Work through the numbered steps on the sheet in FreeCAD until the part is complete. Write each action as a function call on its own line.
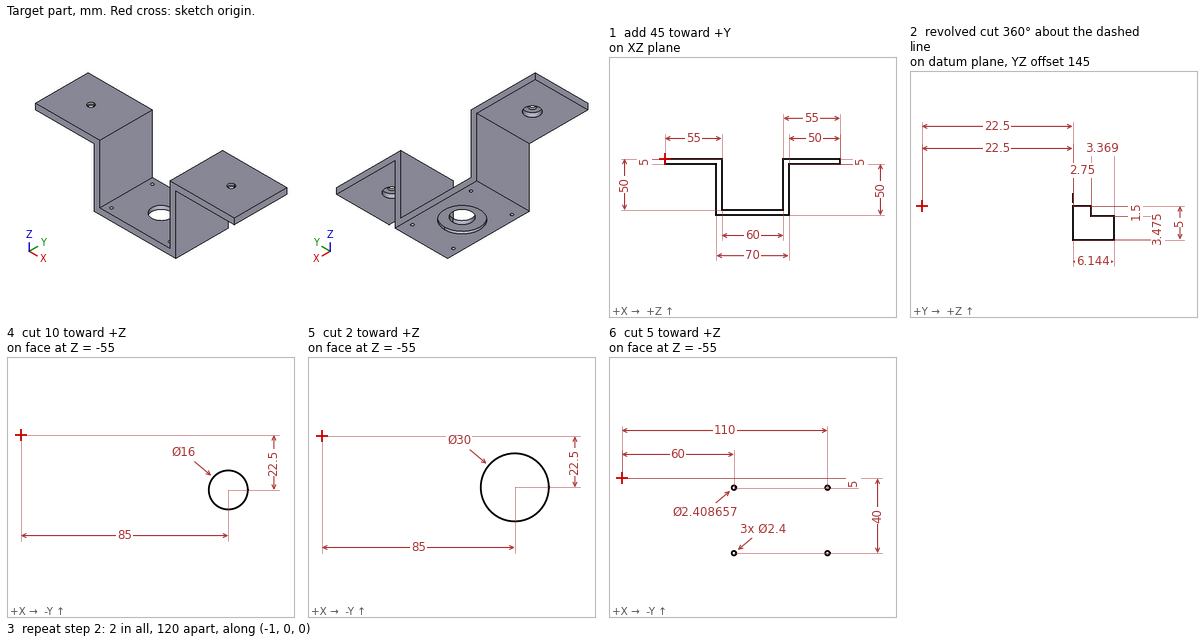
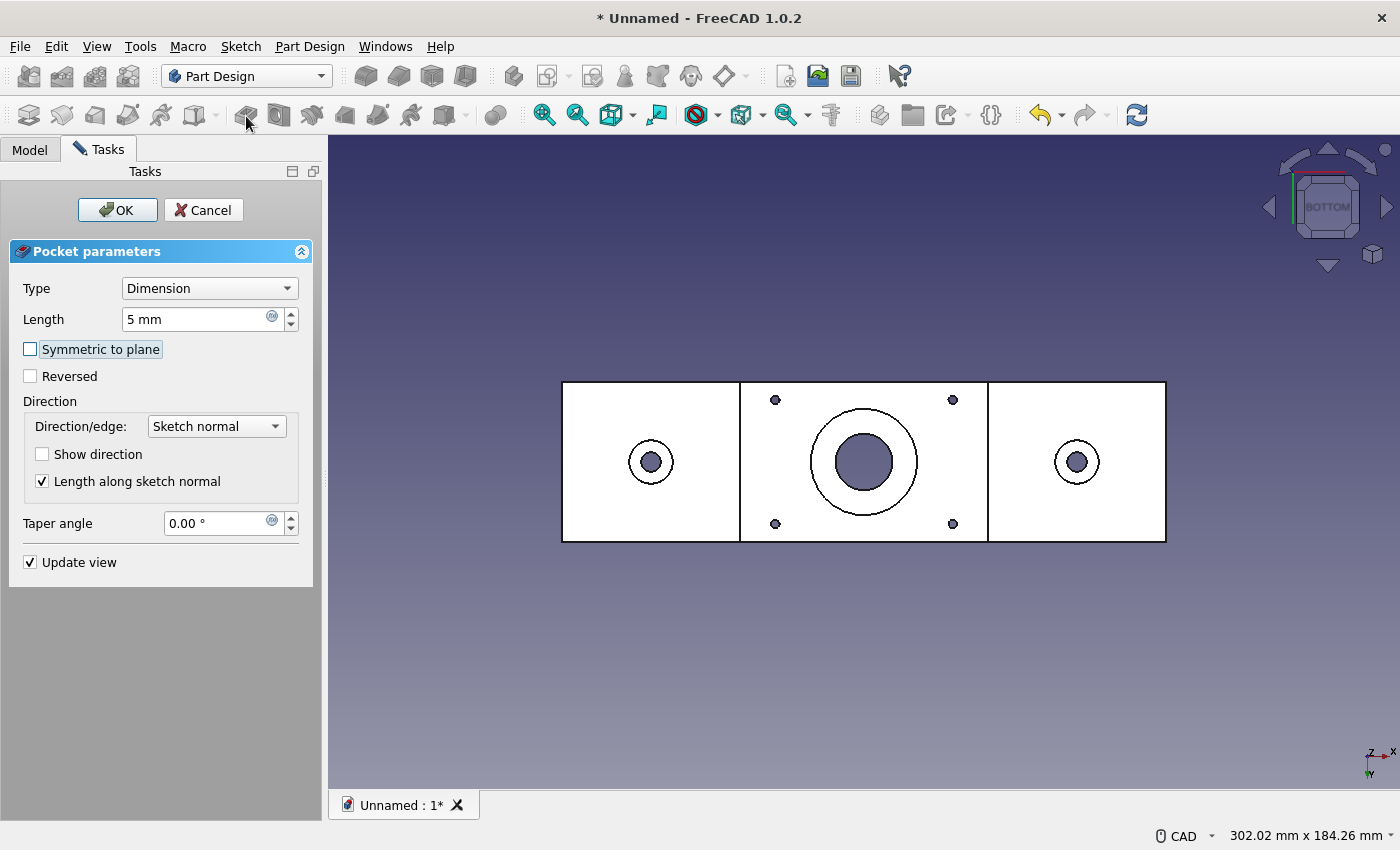
click(118, 210)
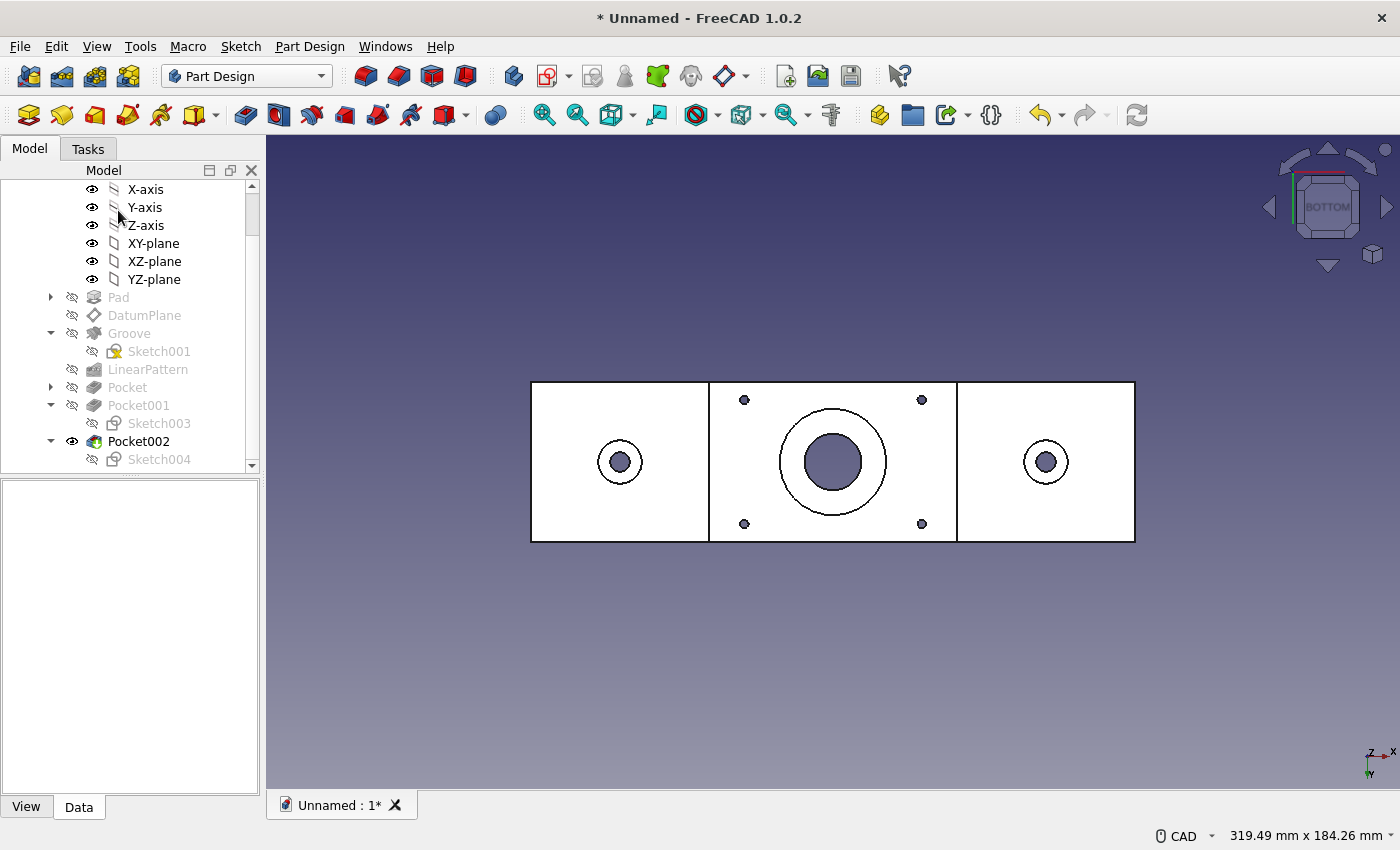
key(0)